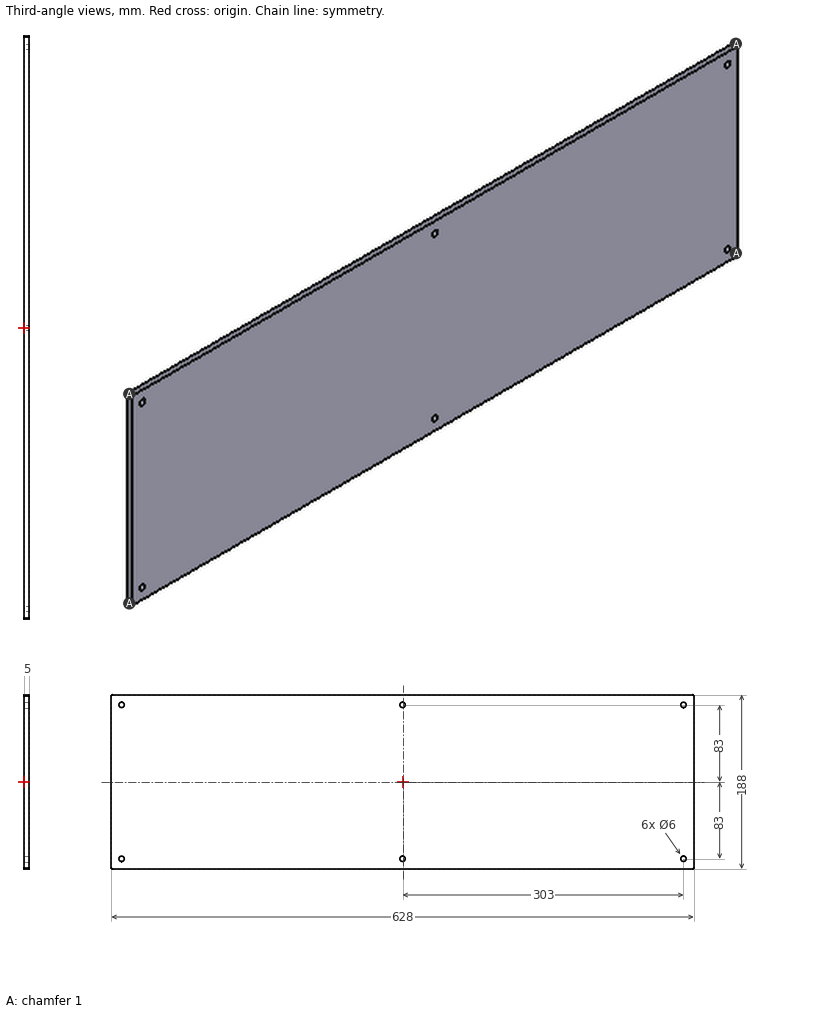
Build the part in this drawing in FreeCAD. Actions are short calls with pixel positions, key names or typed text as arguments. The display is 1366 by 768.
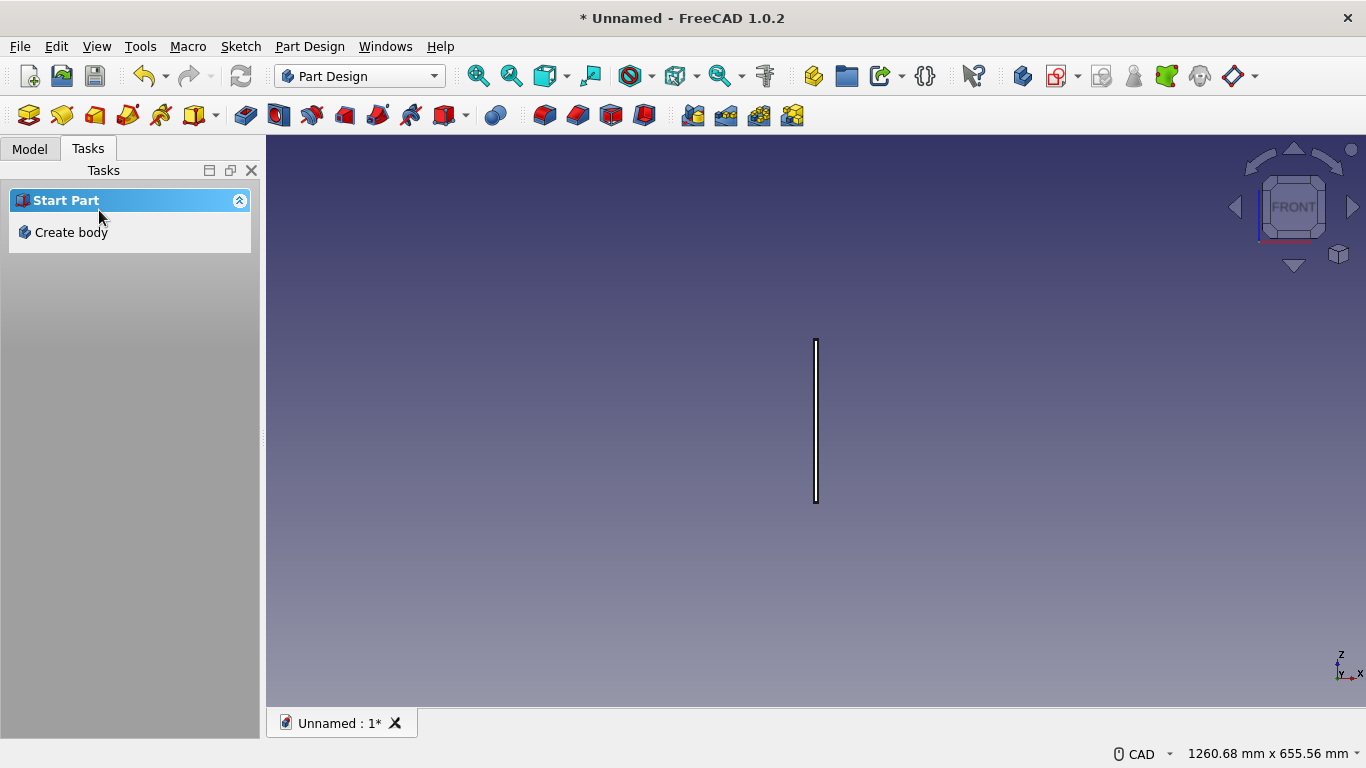
key(6)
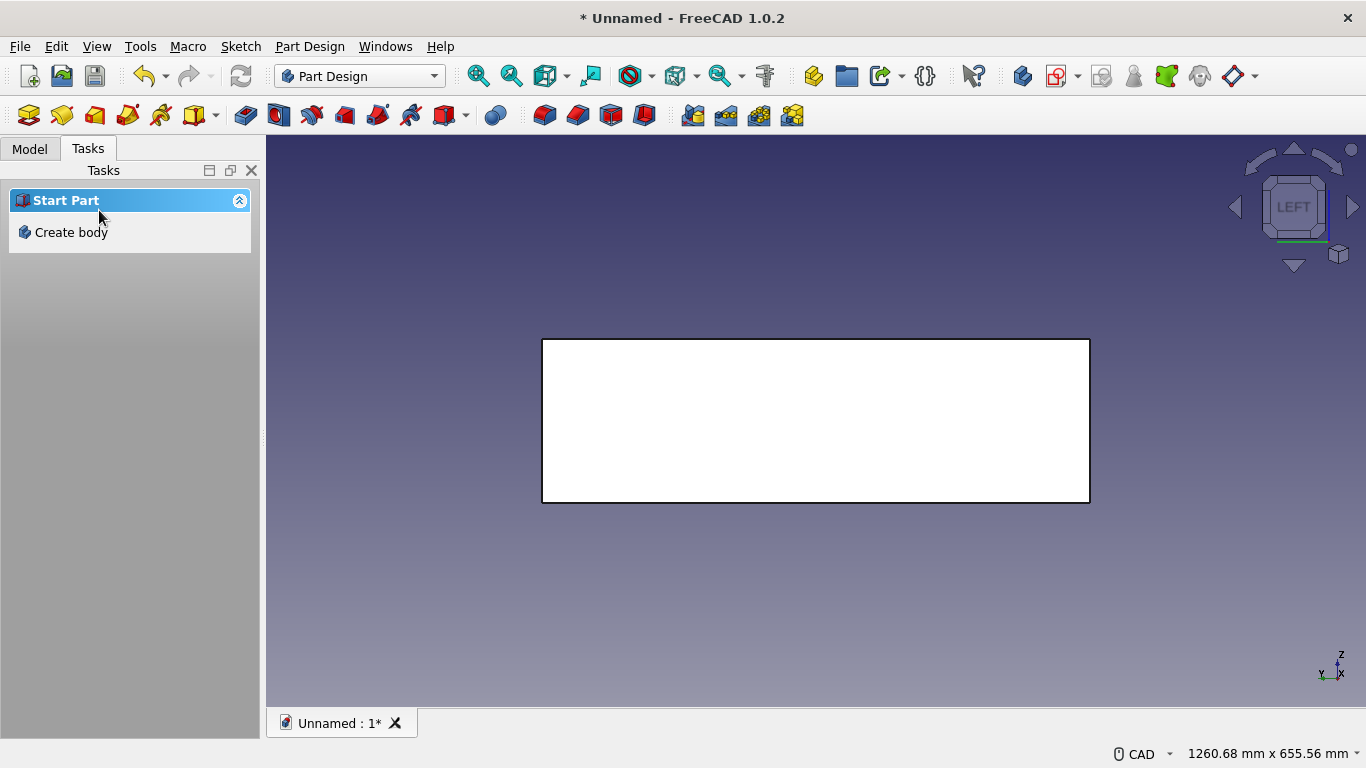
click(659, 420)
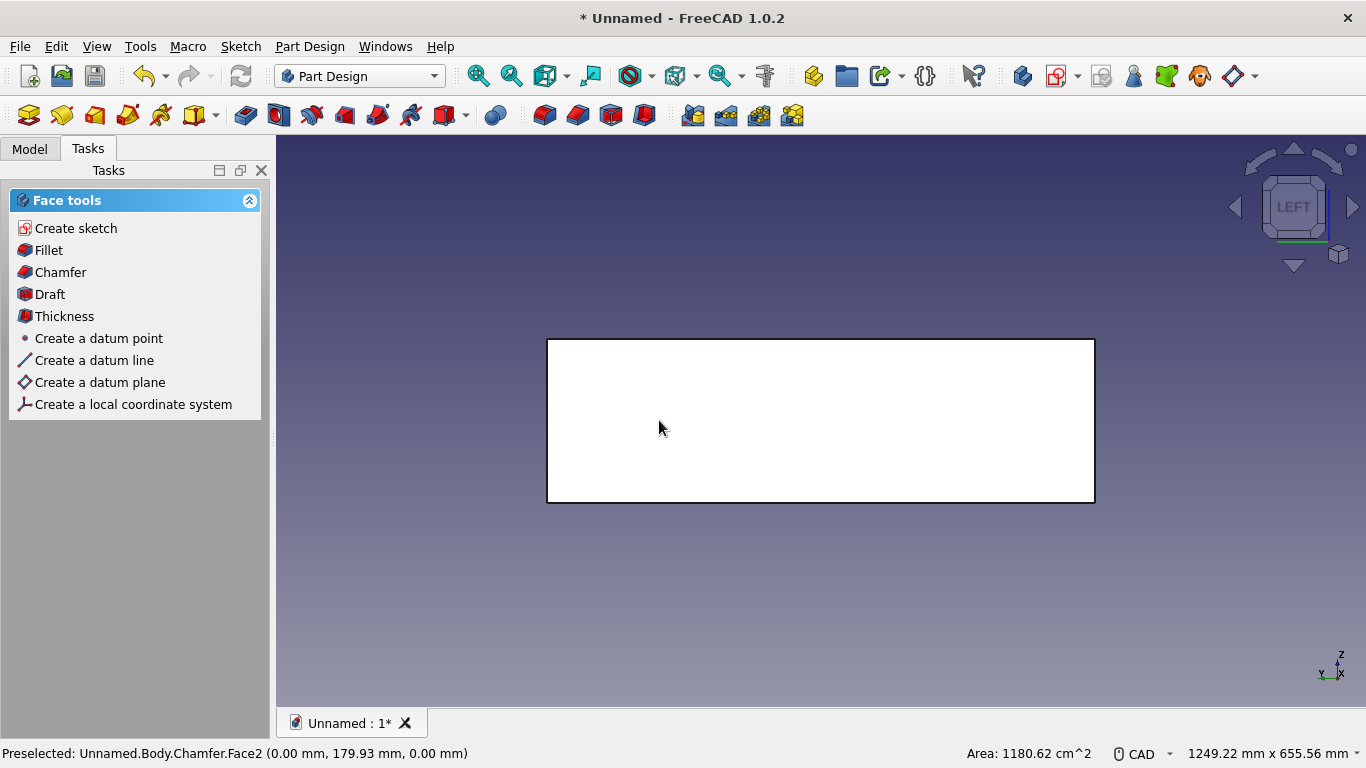
click(1056, 76)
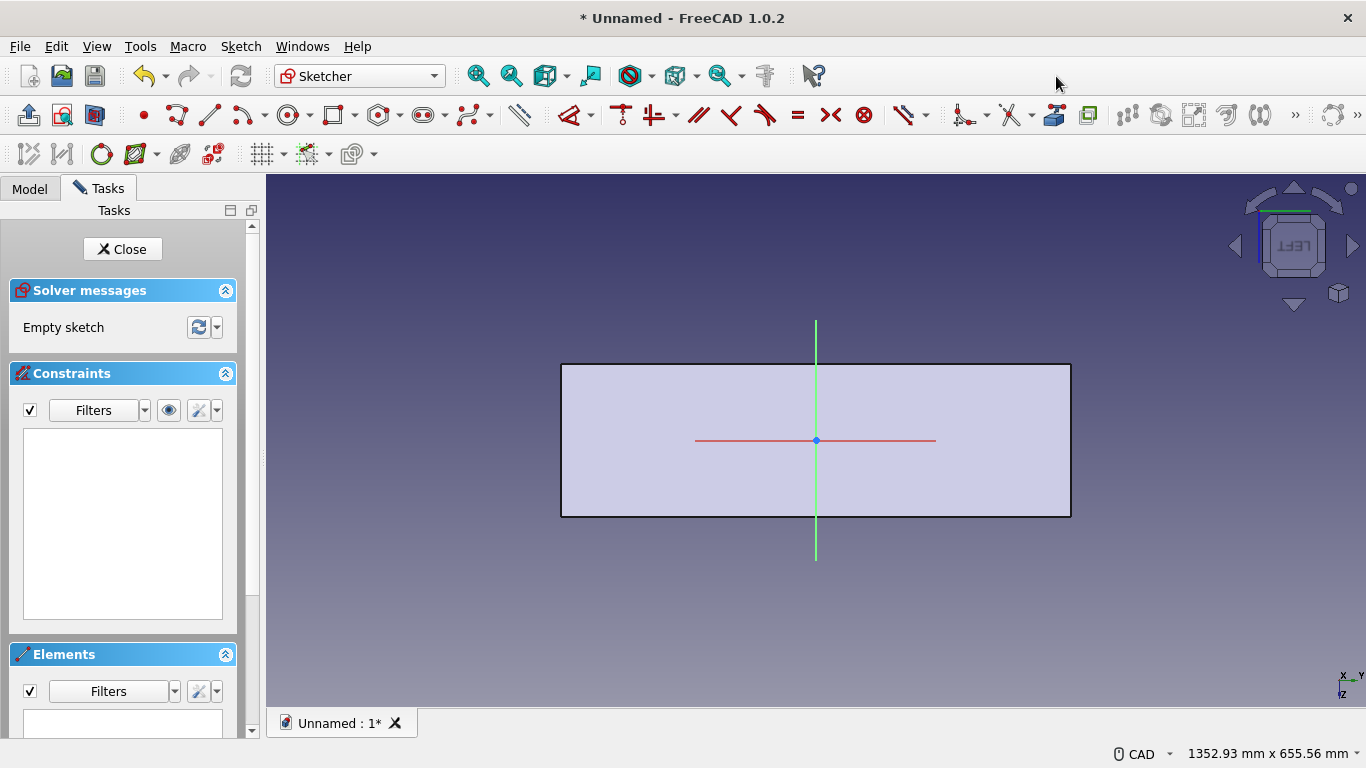
click(288, 116)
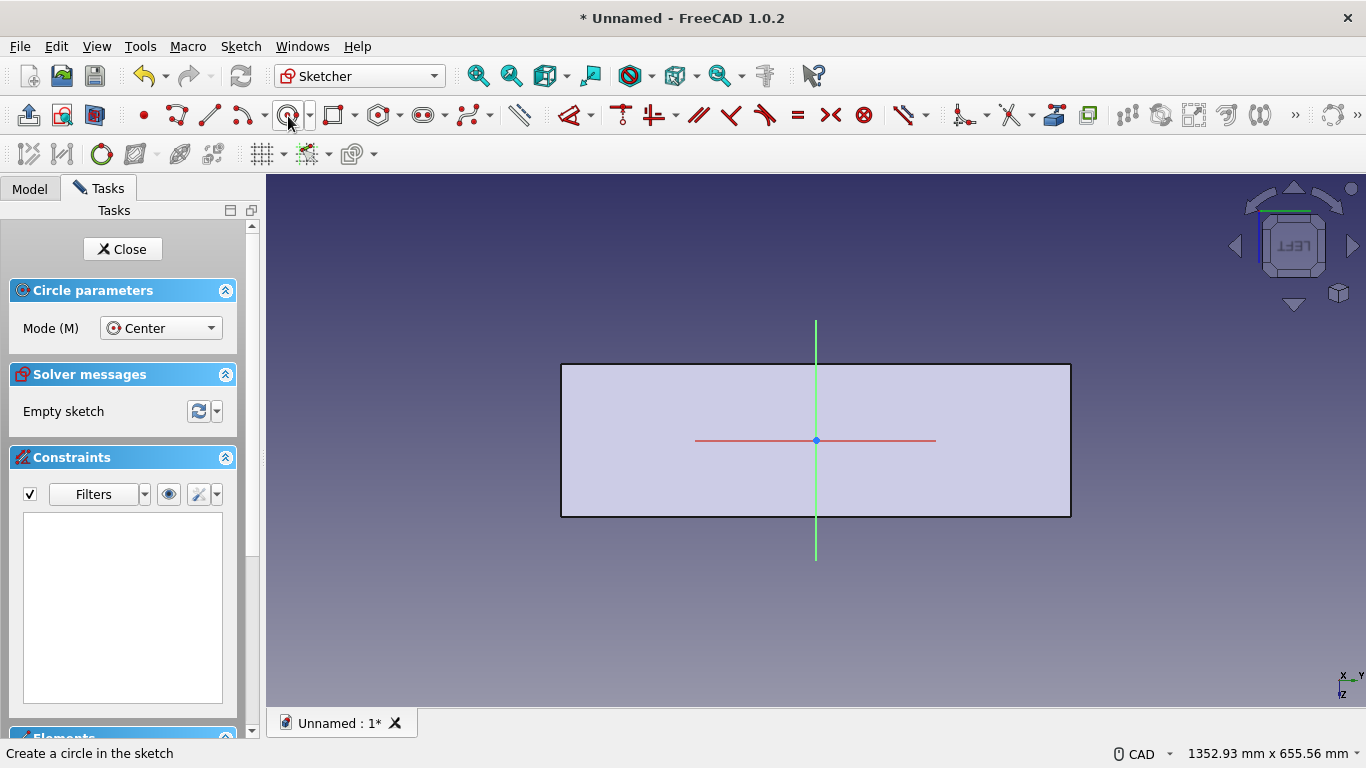
scroll(1062, 373, up, 12)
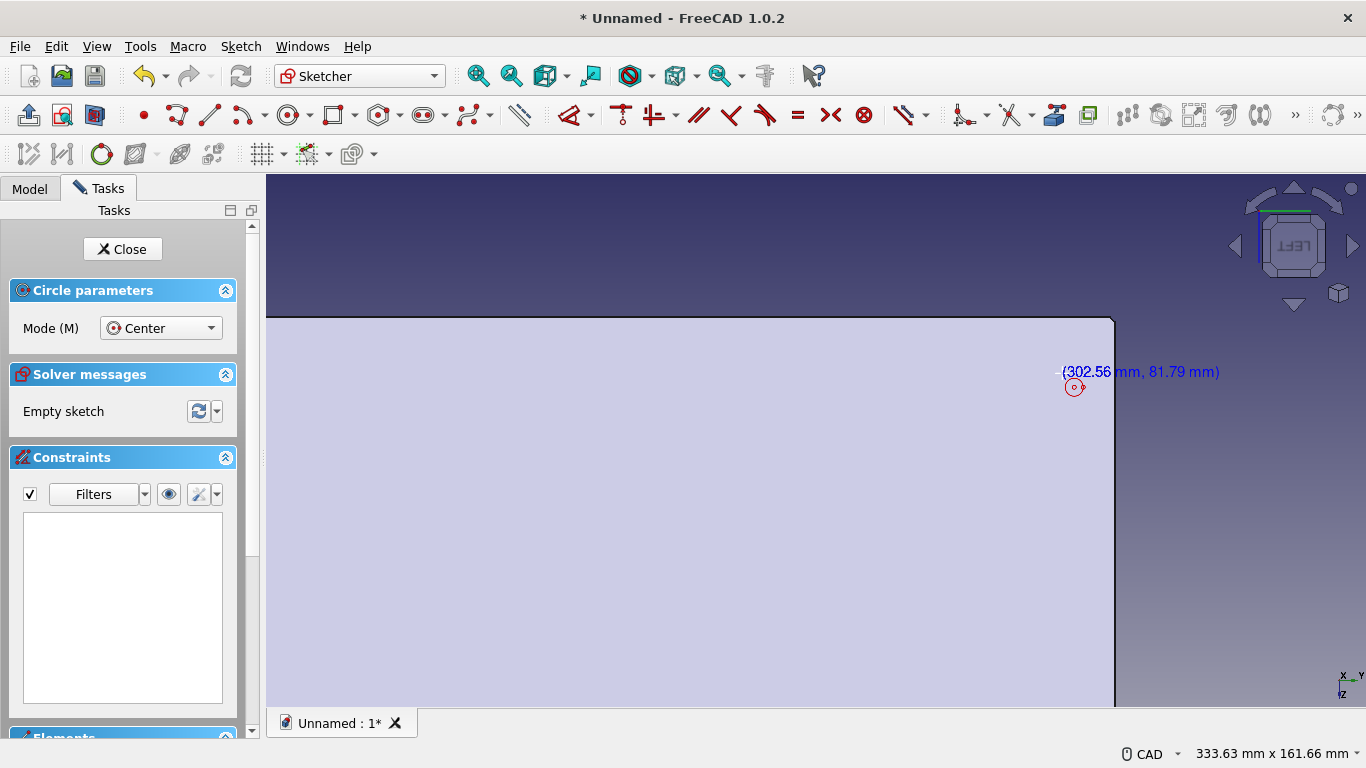
scroll(1047, 357, down, 11)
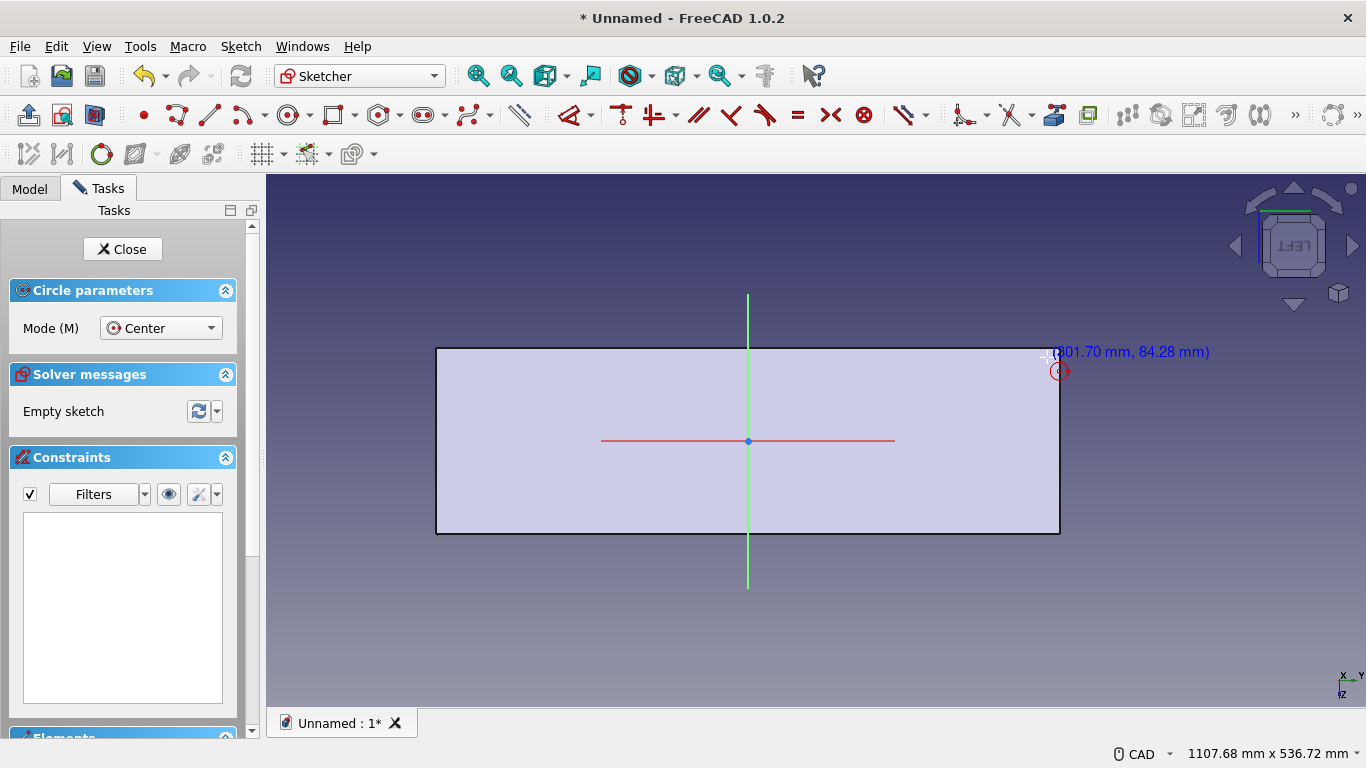
click(1049, 359)
move(1051, 357)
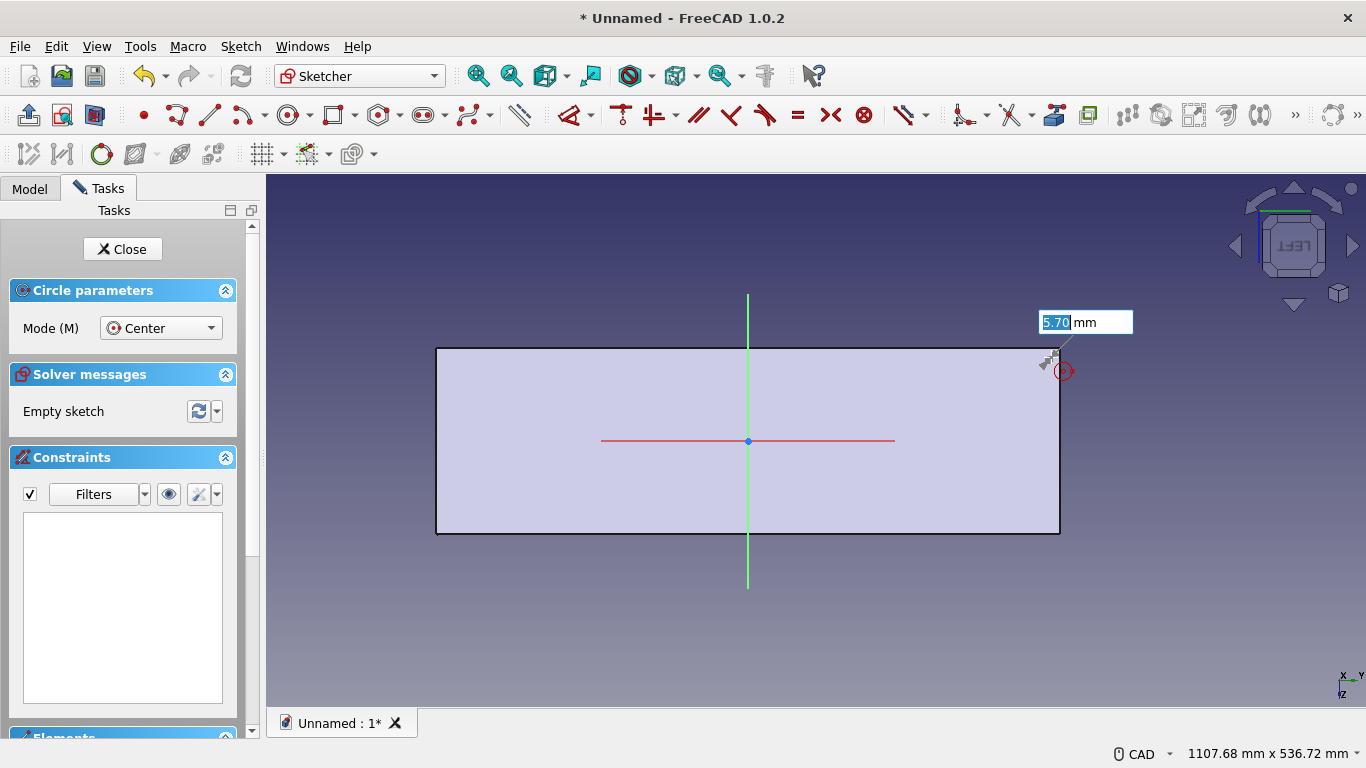
text(6)
key(Return)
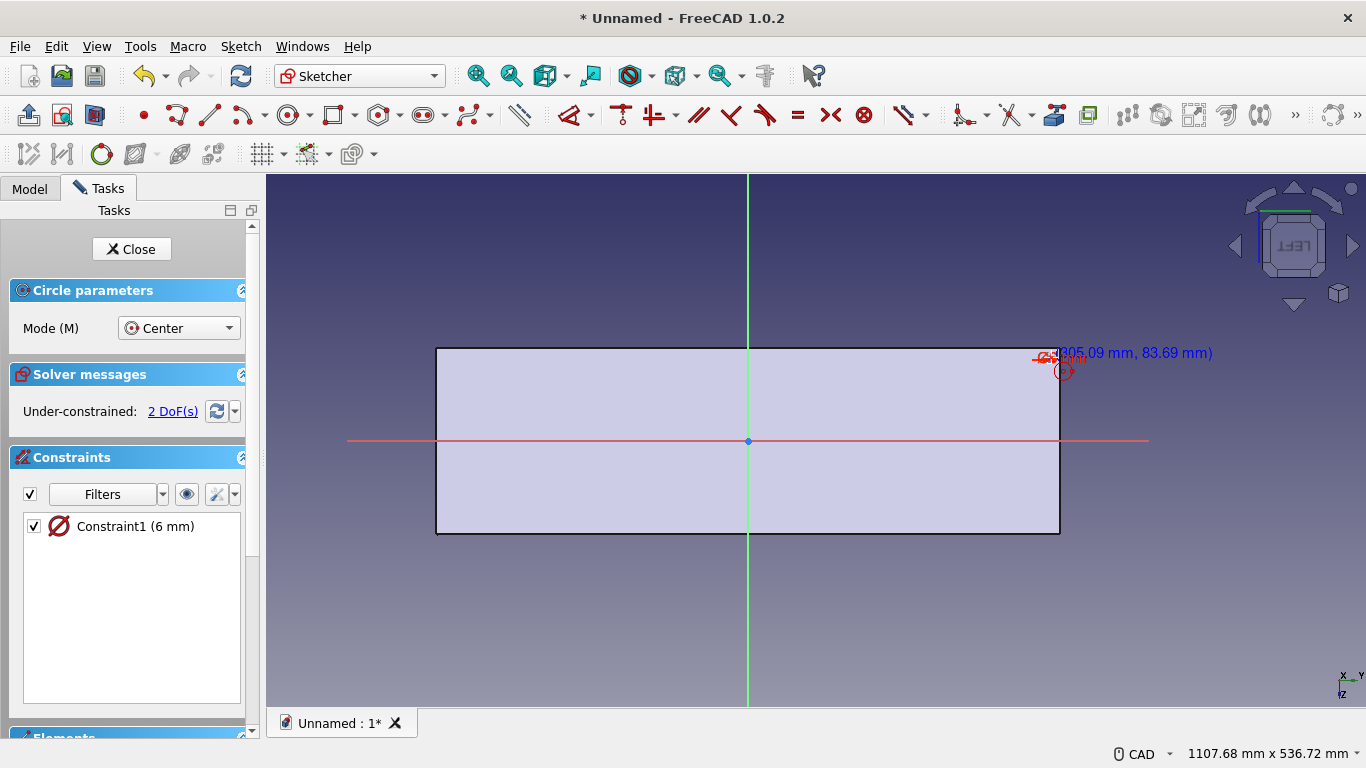
scroll(447, 359, up, 11)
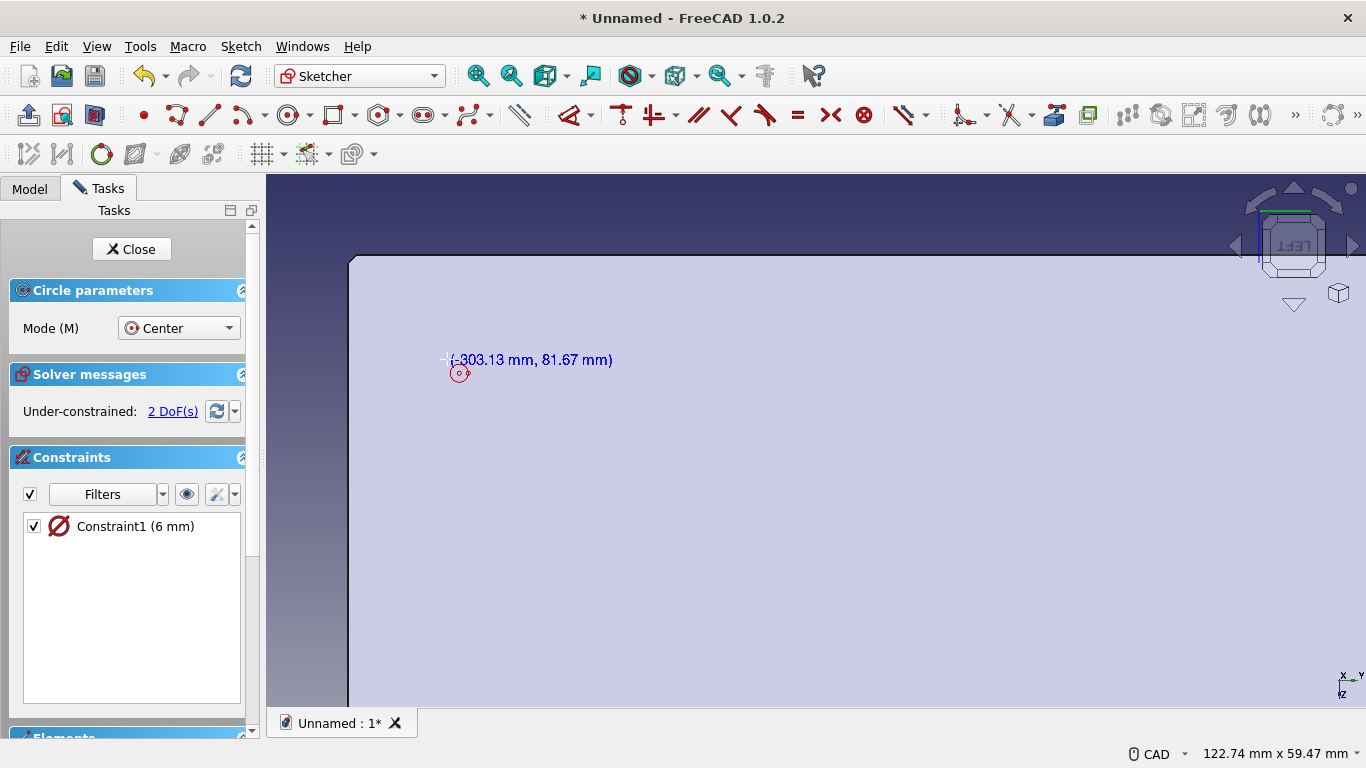
scroll(447, 359, down, 11)